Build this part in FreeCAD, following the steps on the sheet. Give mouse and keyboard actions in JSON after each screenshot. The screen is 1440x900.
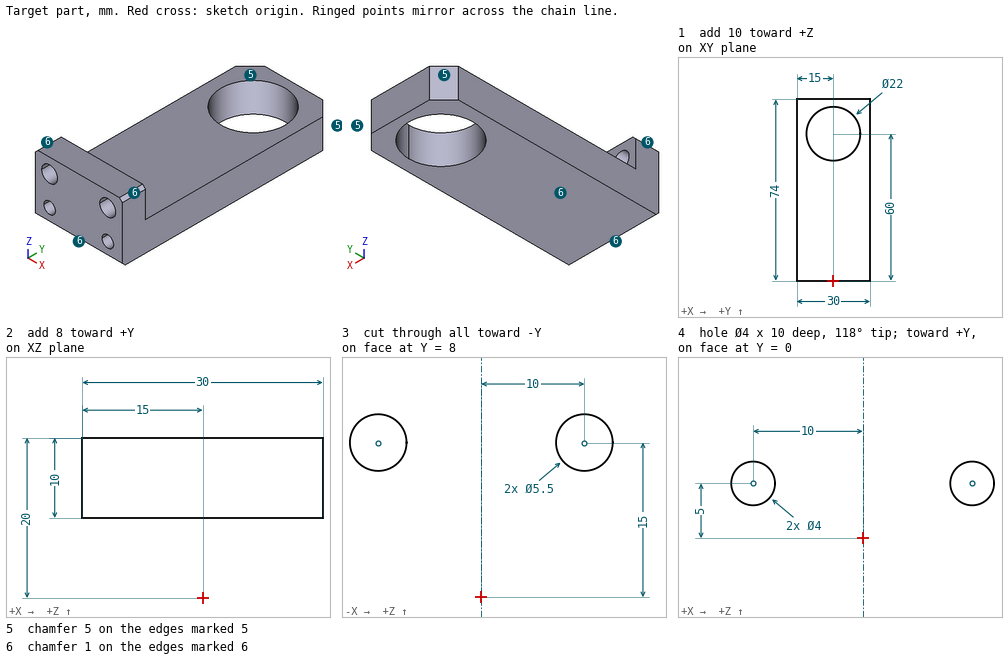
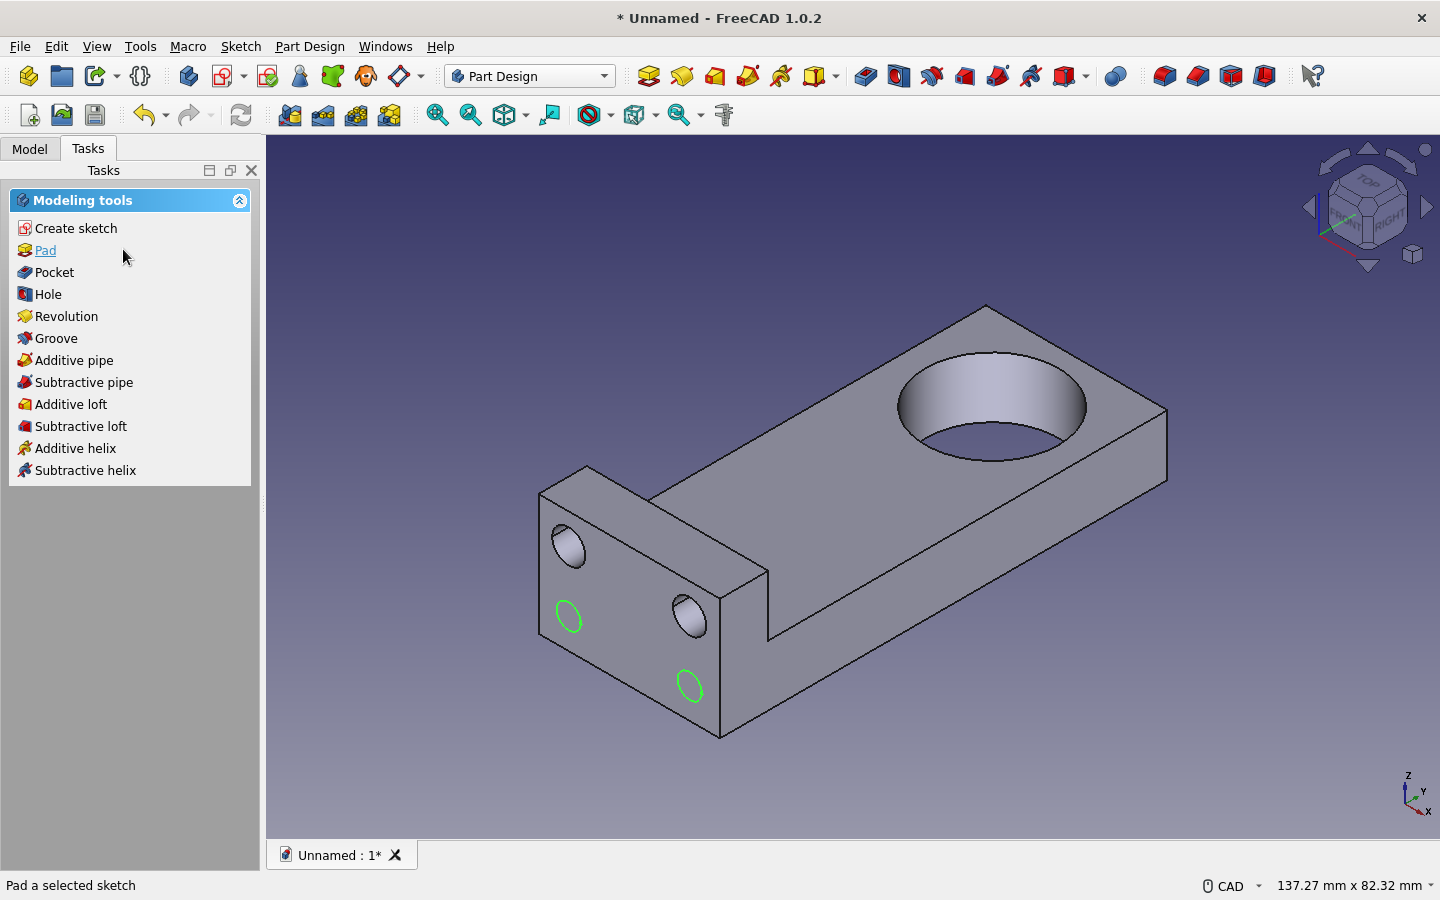
{"action": "left_click", "coordinate": [899, 76]}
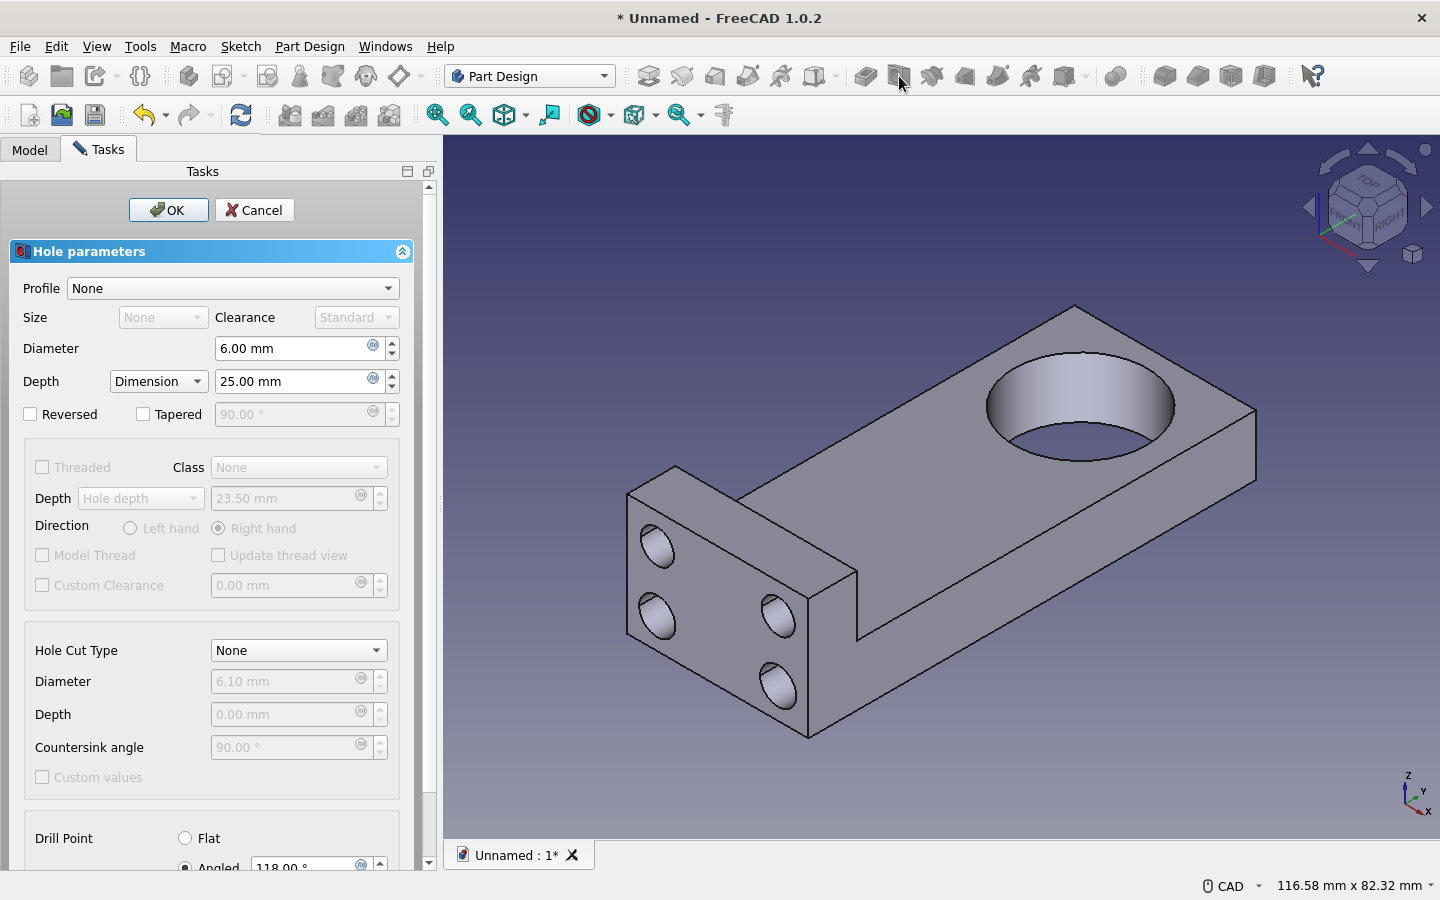
{"action": "triple_click", "coordinate": [300, 348]}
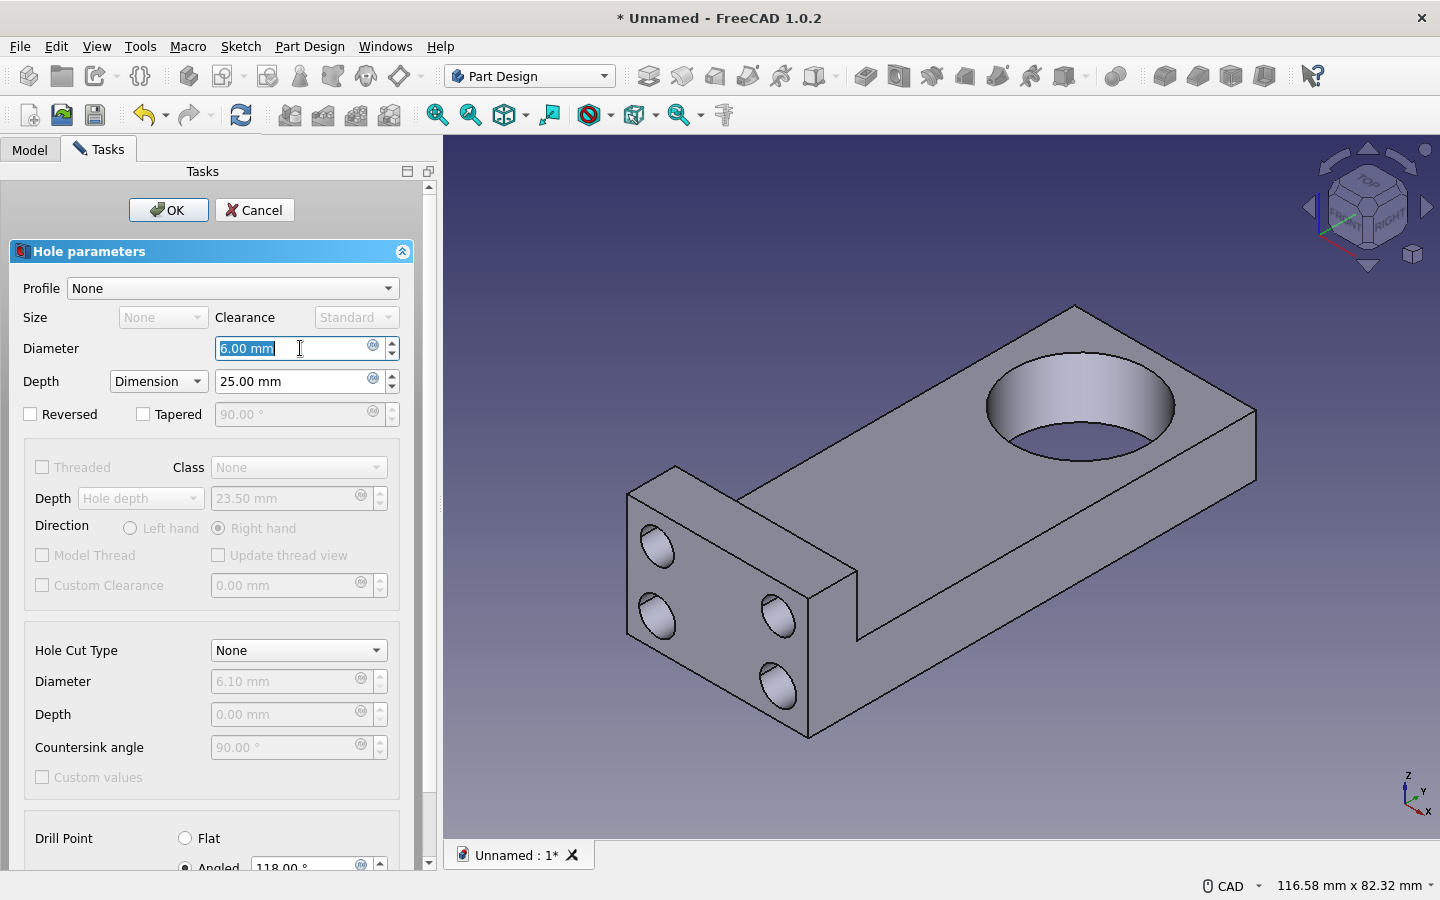
{"action": "type", "text": "4"}
{"action": "key", "text": "Tab"}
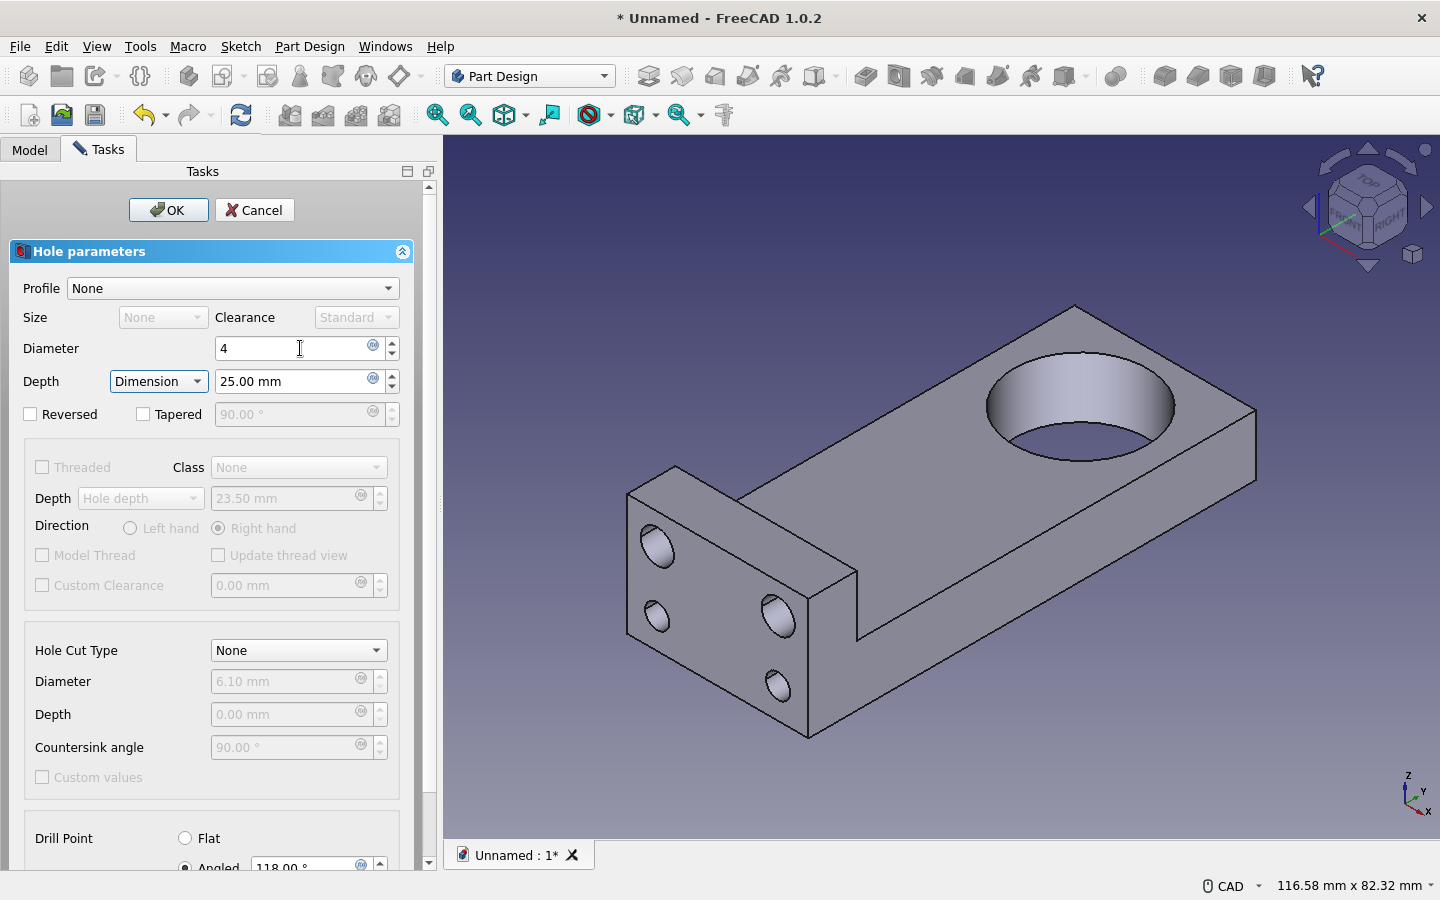
{"action": "triple_click", "coordinate": [300, 382]}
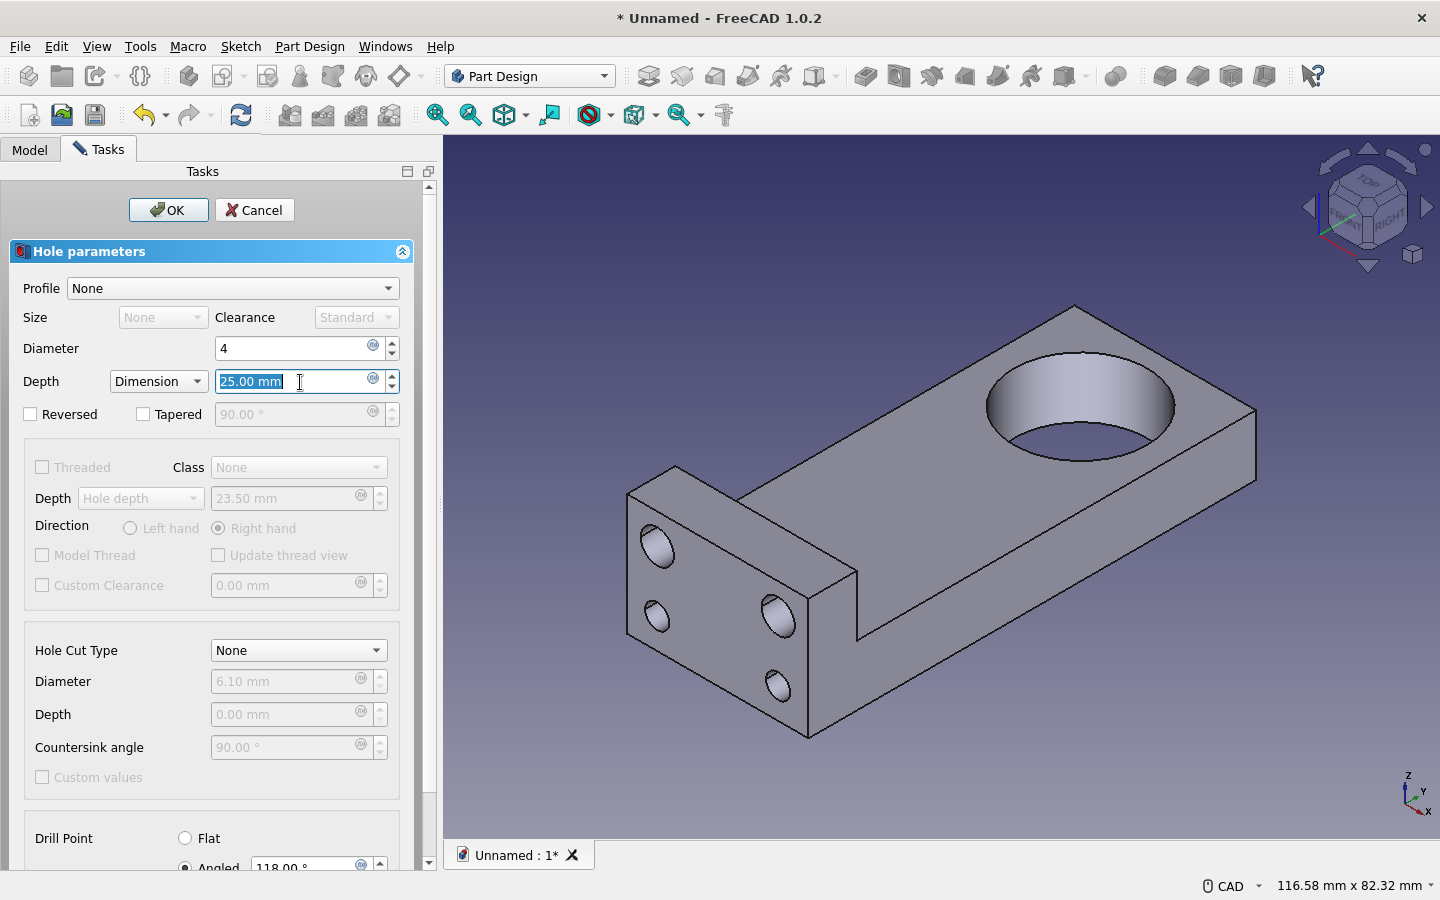
{"action": "type", "text": "10"}
{"action": "key", "text": "Tab"}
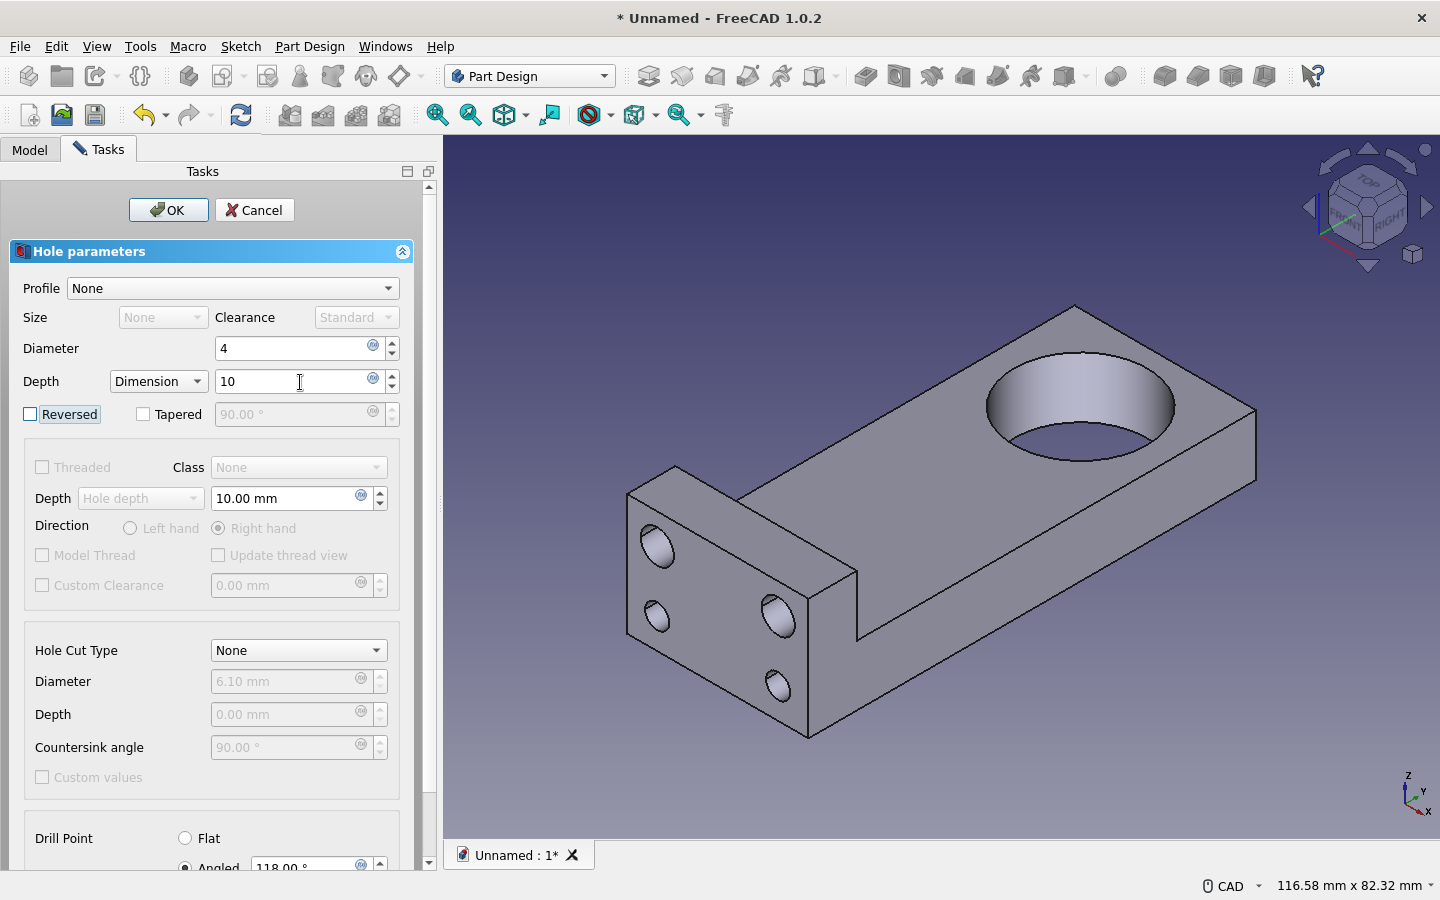
{"action": "left_click", "coordinate": [169, 210]}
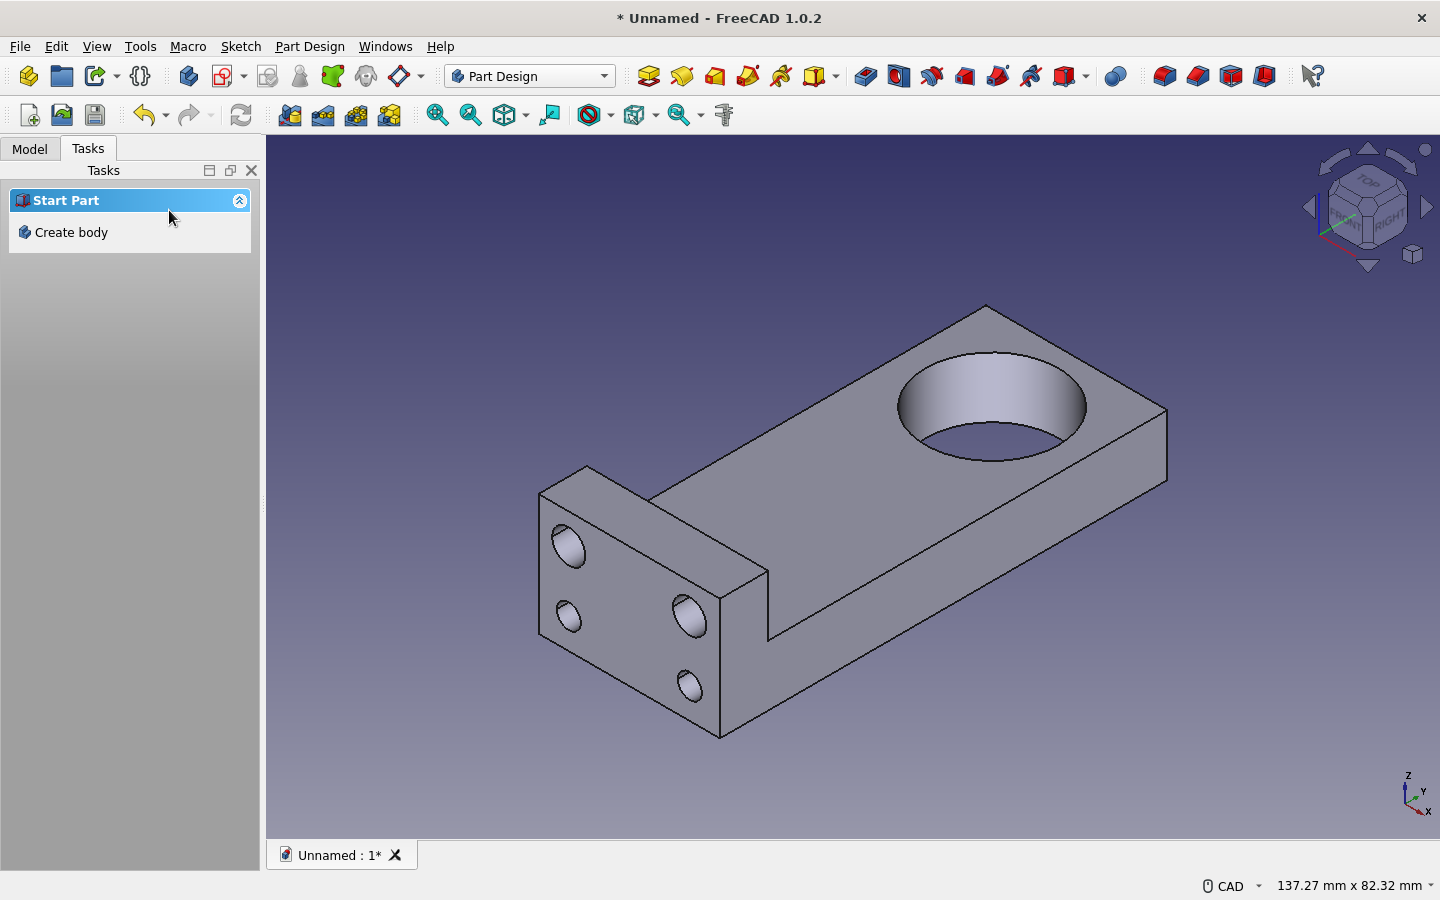
{"action": "key", "text": "2"}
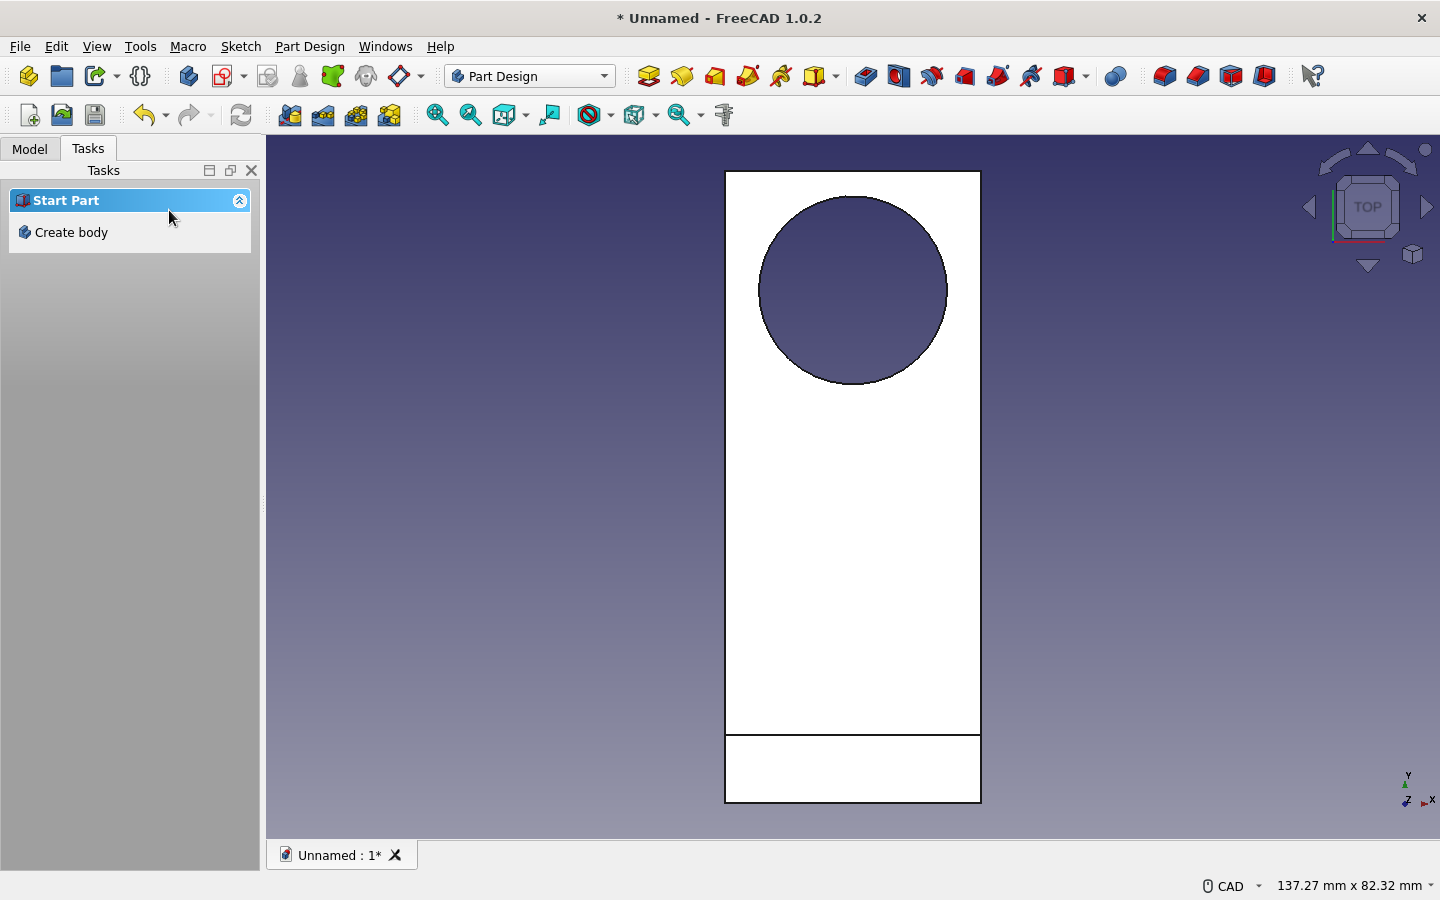
{"action": "key", "text": "0"}